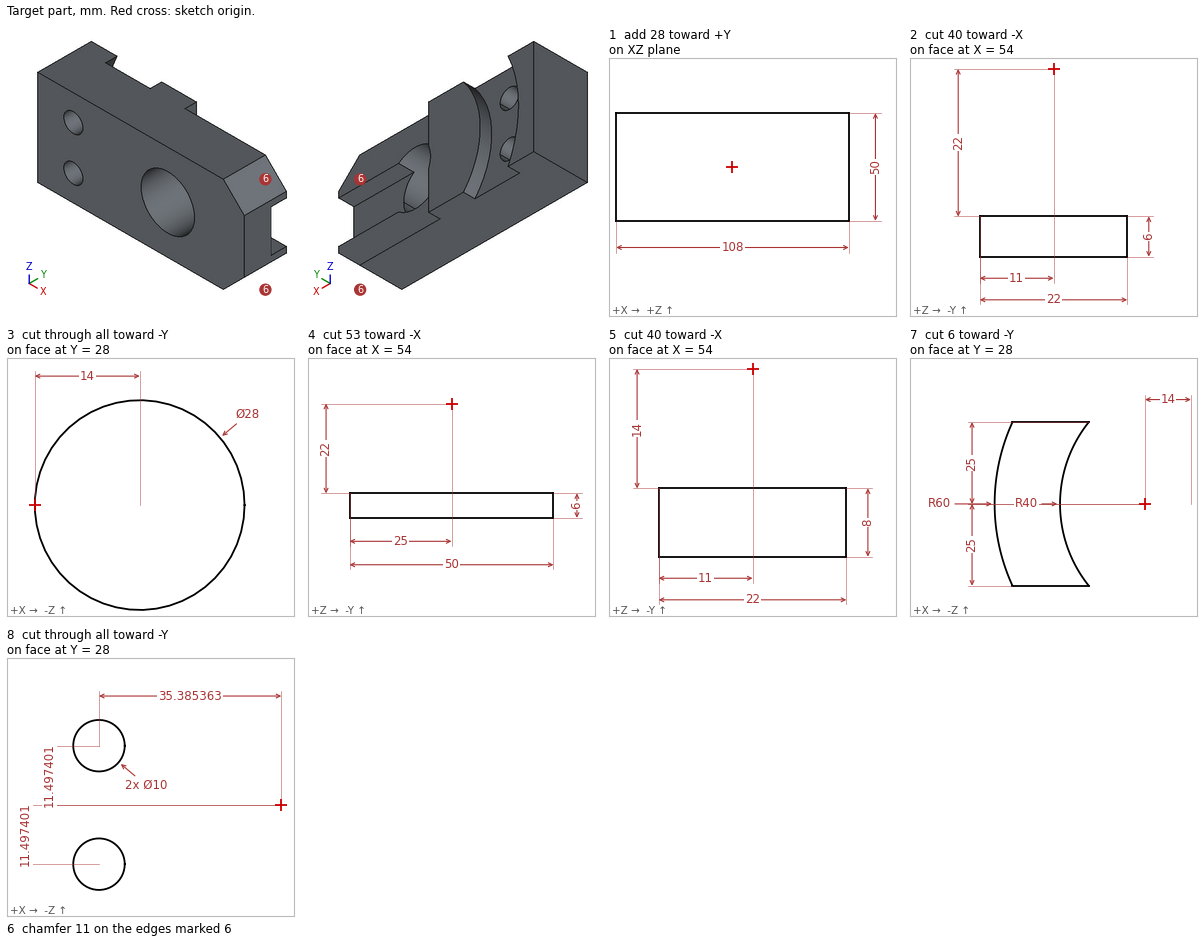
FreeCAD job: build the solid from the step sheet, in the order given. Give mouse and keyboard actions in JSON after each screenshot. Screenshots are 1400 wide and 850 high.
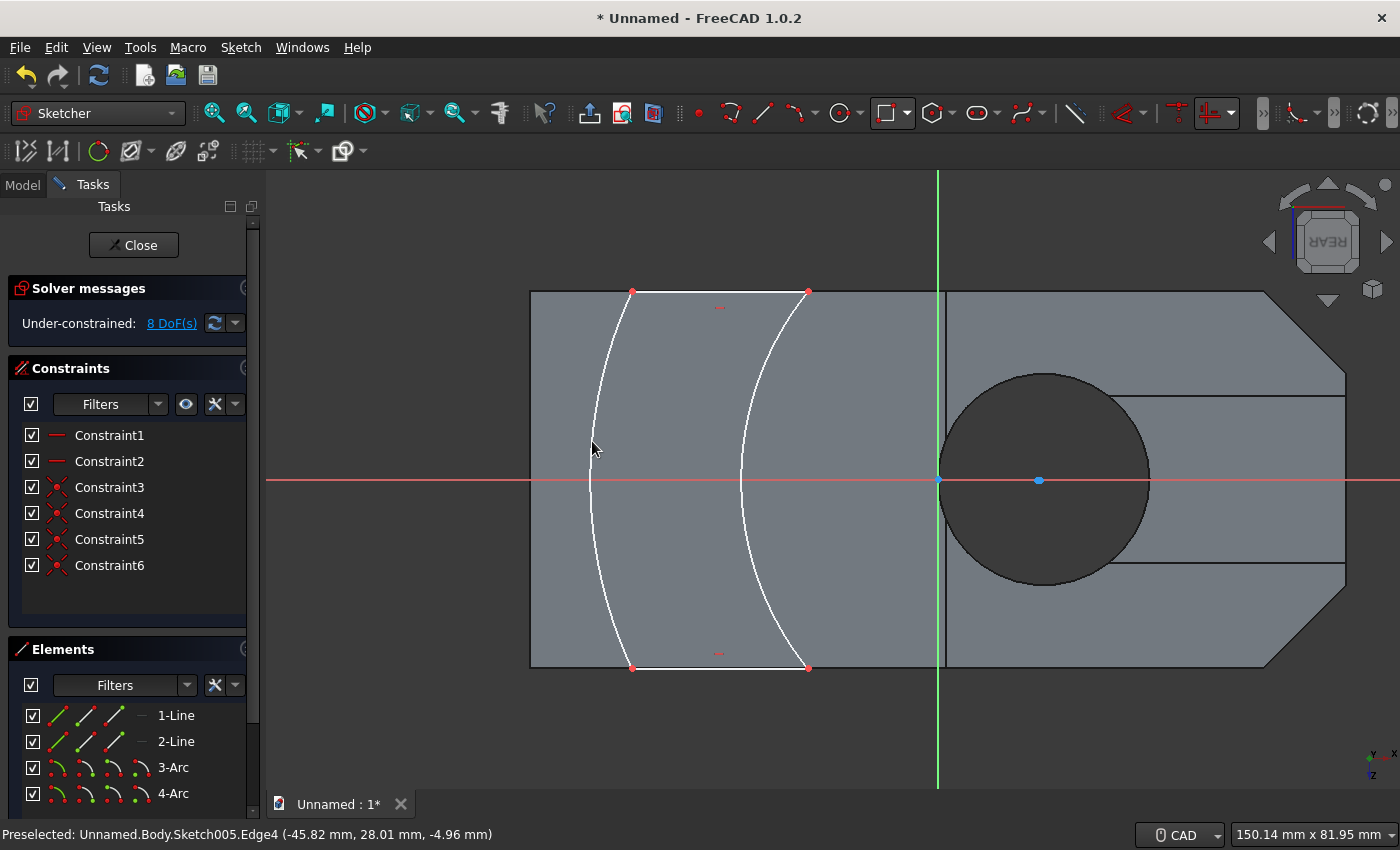
{"action": "left_click", "coordinate": [752, 400]}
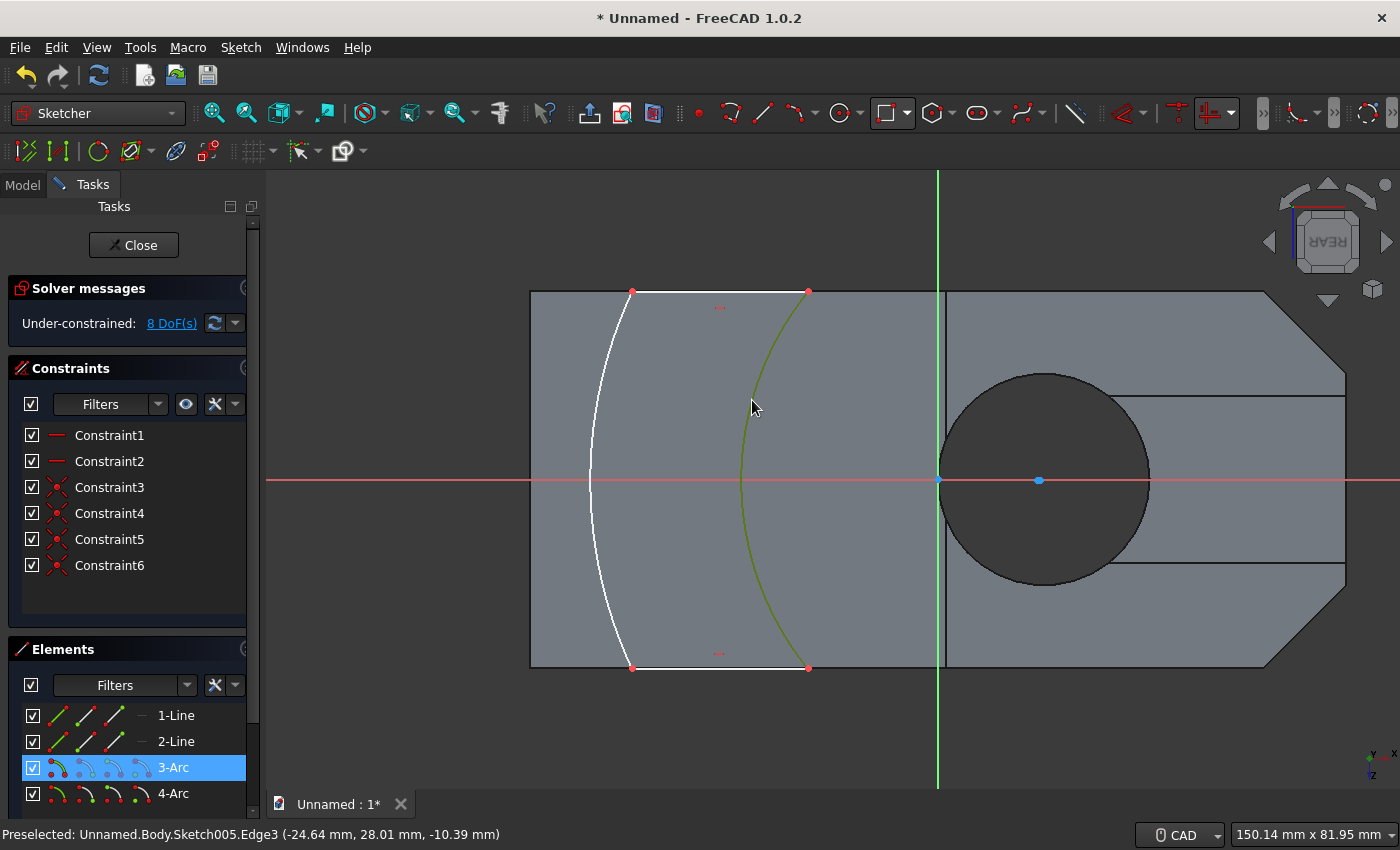
{"action": "left_click", "coordinate": [597, 403]}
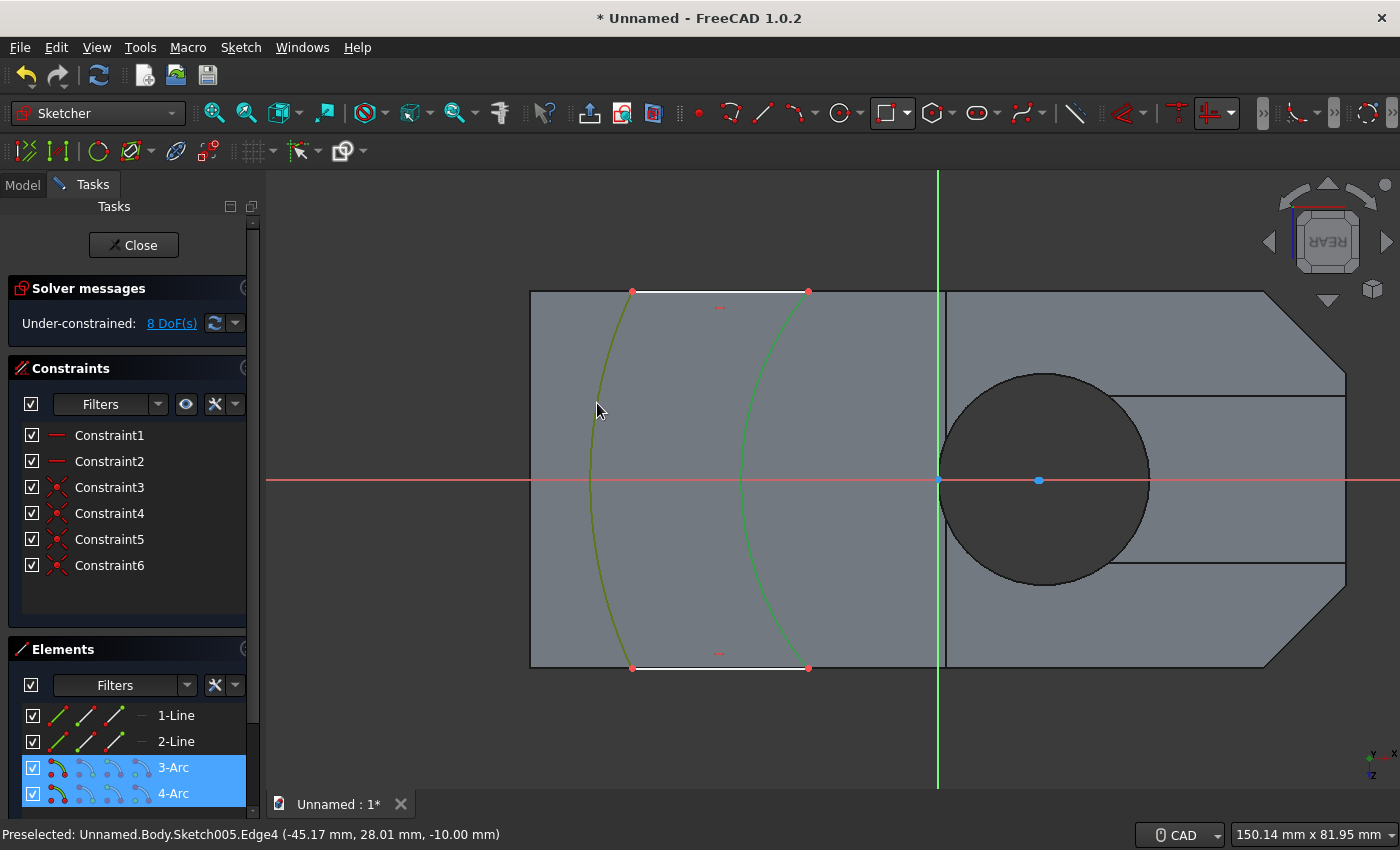
{"action": "key", "text": "c"}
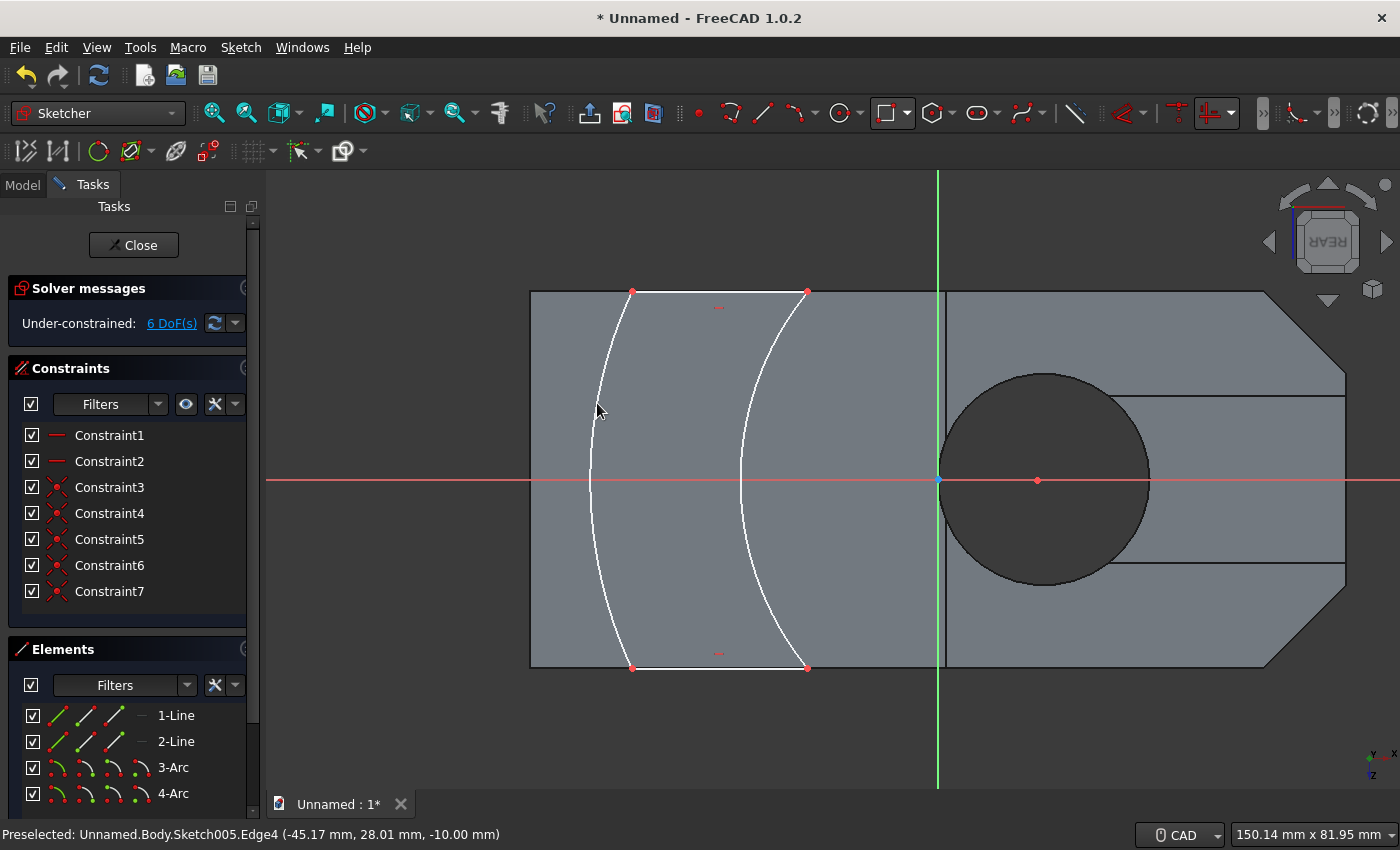
{"action": "left_click", "coordinate": [1038, 481]}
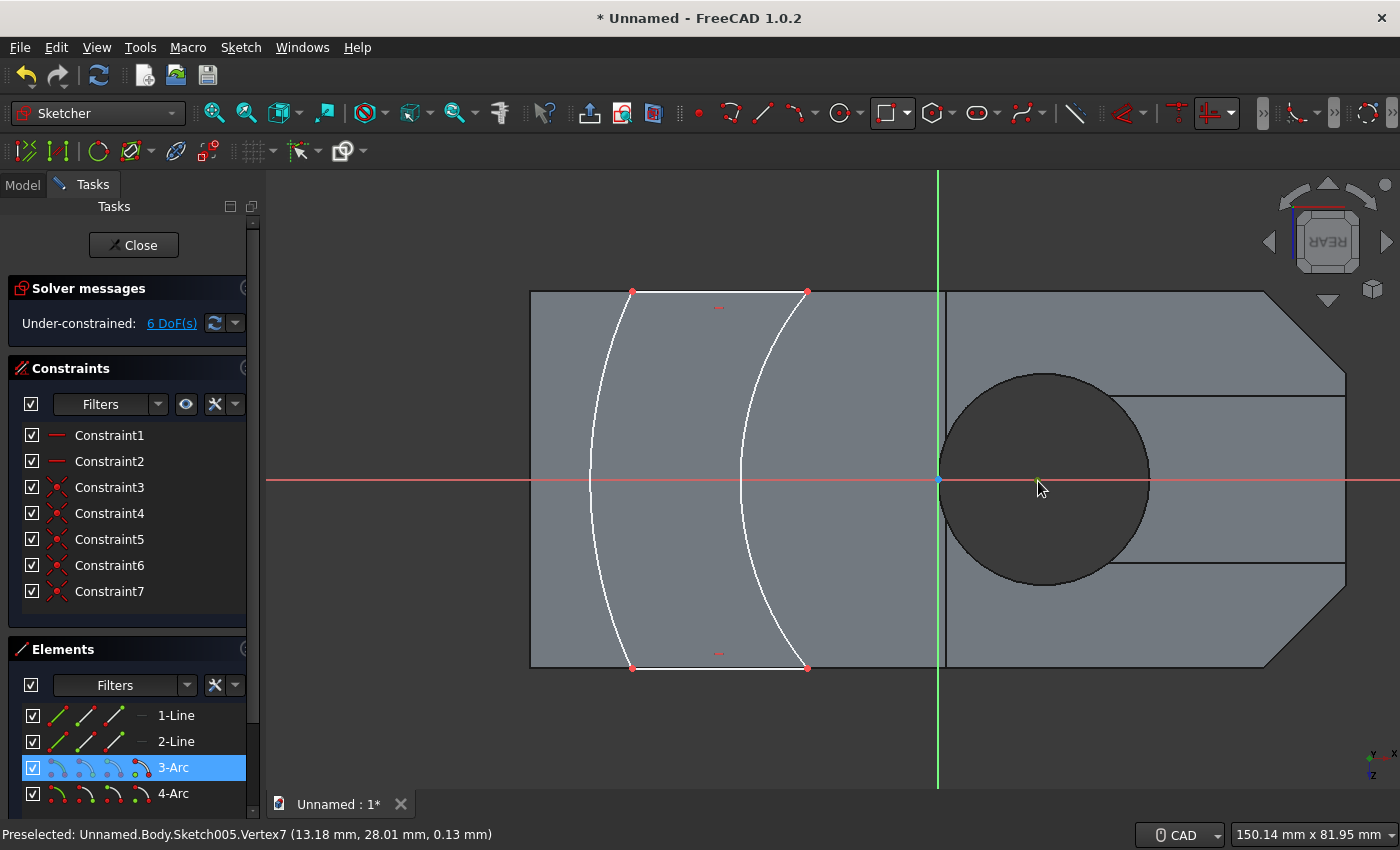
{"action": "left_click", "coordinate": [361, 479]}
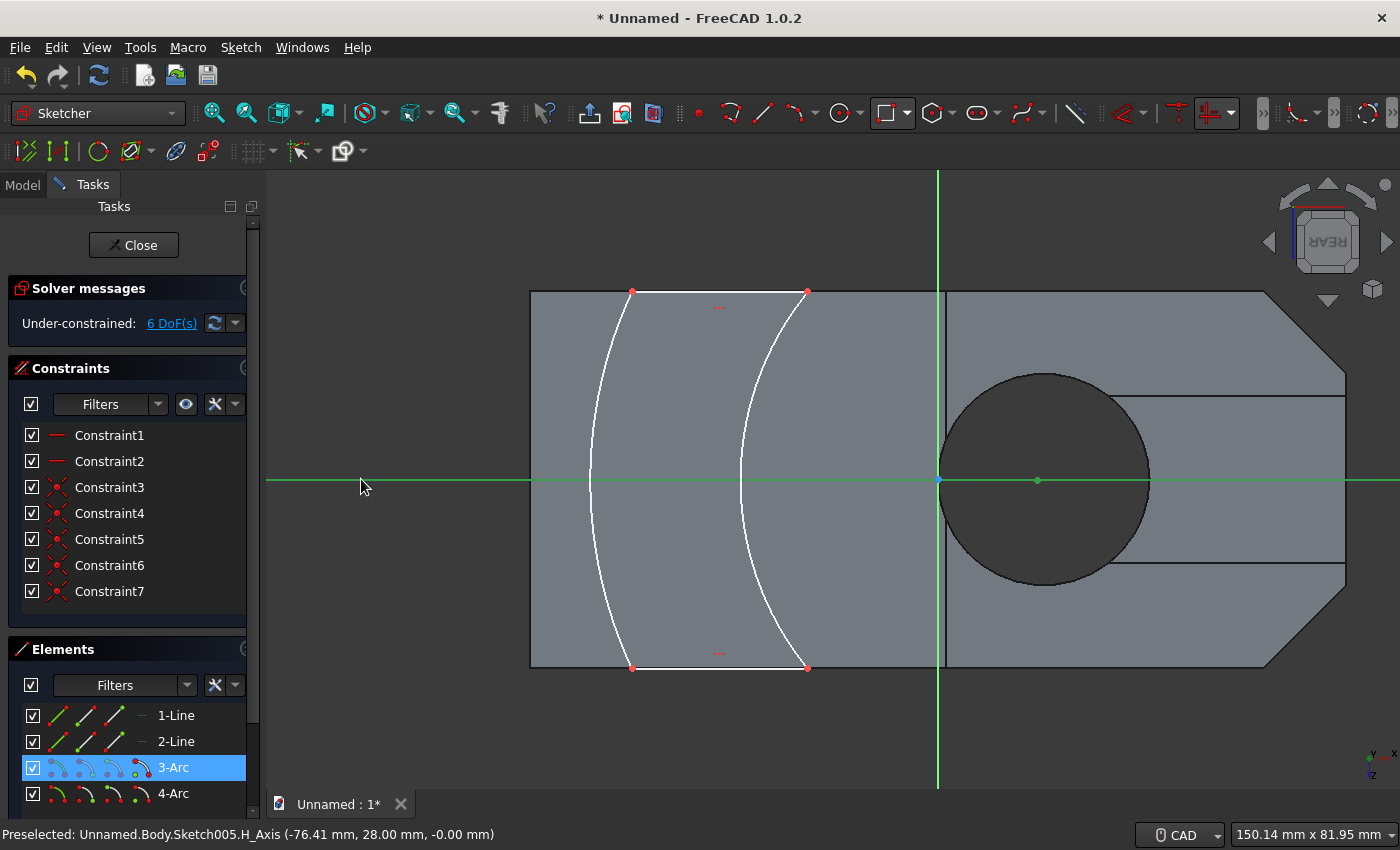
{"action": "left_click", "coordinate": [1178, 114]}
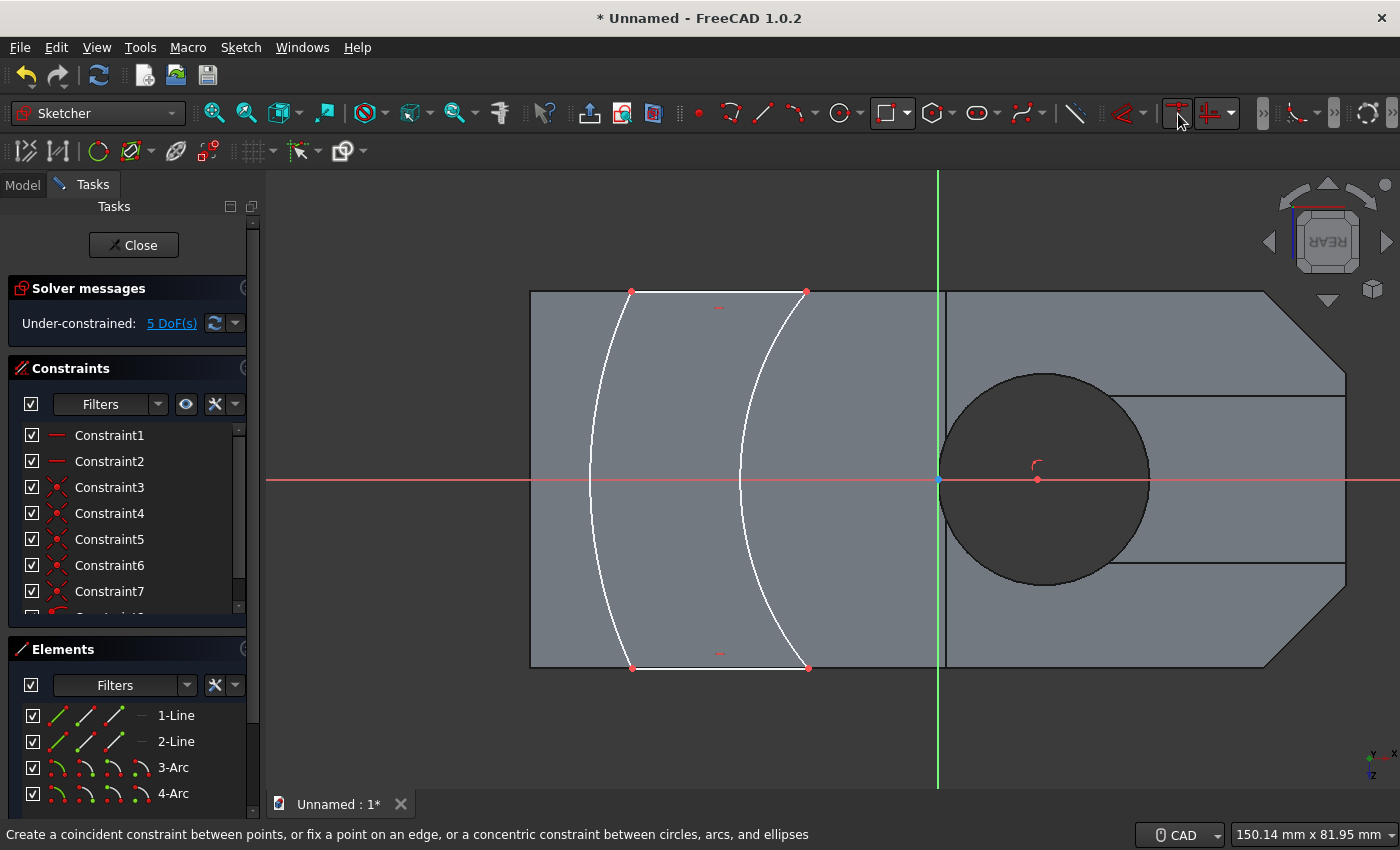
{"action": "key", "text": "d"}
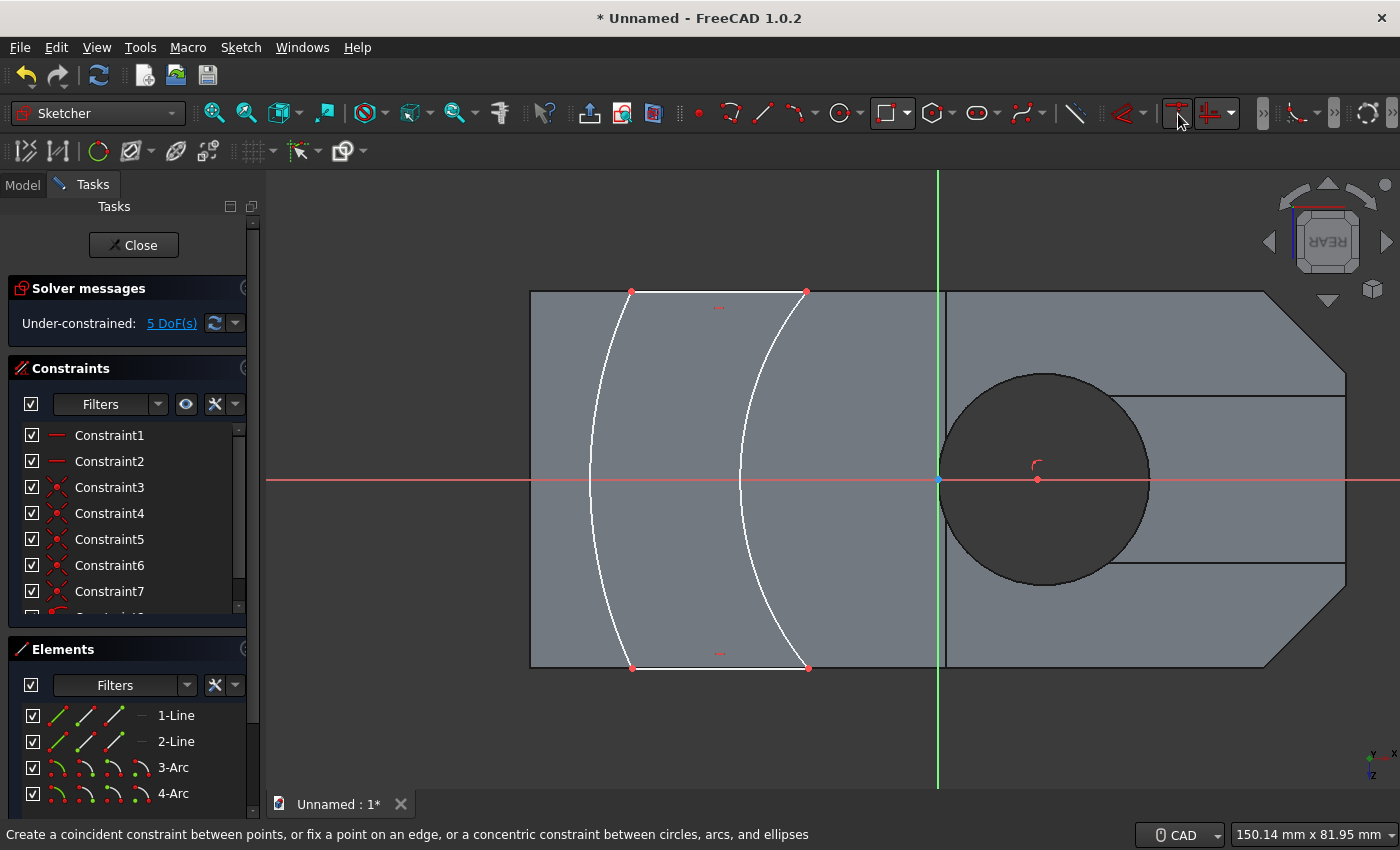
{"action": "left_click", "coordinate": [751, 400]}
{"action": "left_click", "coordinate": [720, 391]}